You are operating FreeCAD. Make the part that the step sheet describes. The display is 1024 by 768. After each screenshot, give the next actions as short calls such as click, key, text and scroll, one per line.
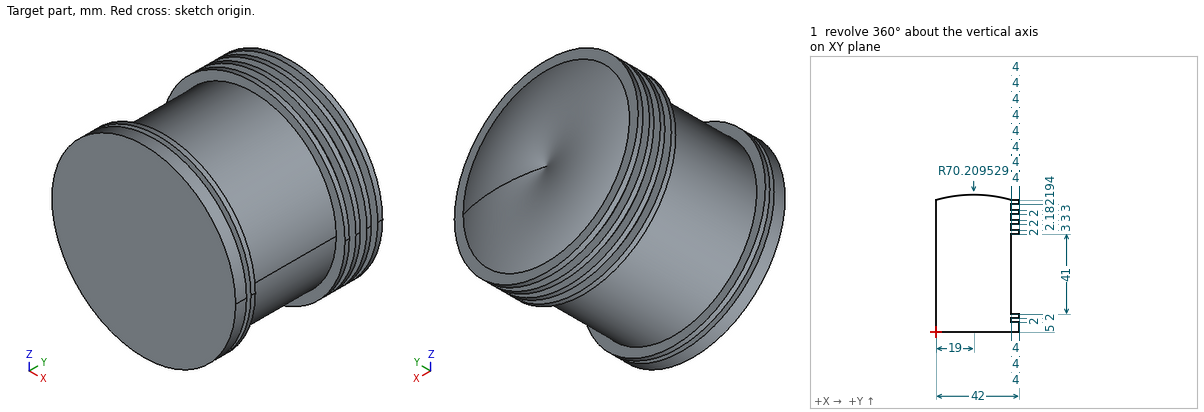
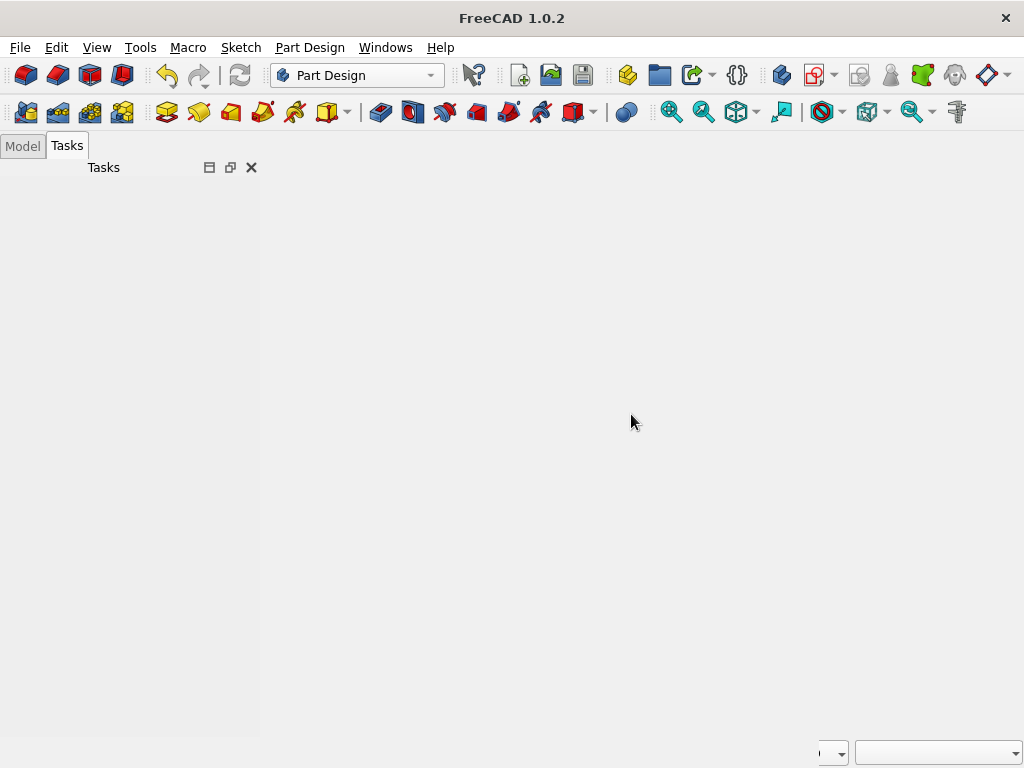
key(ctrl+n)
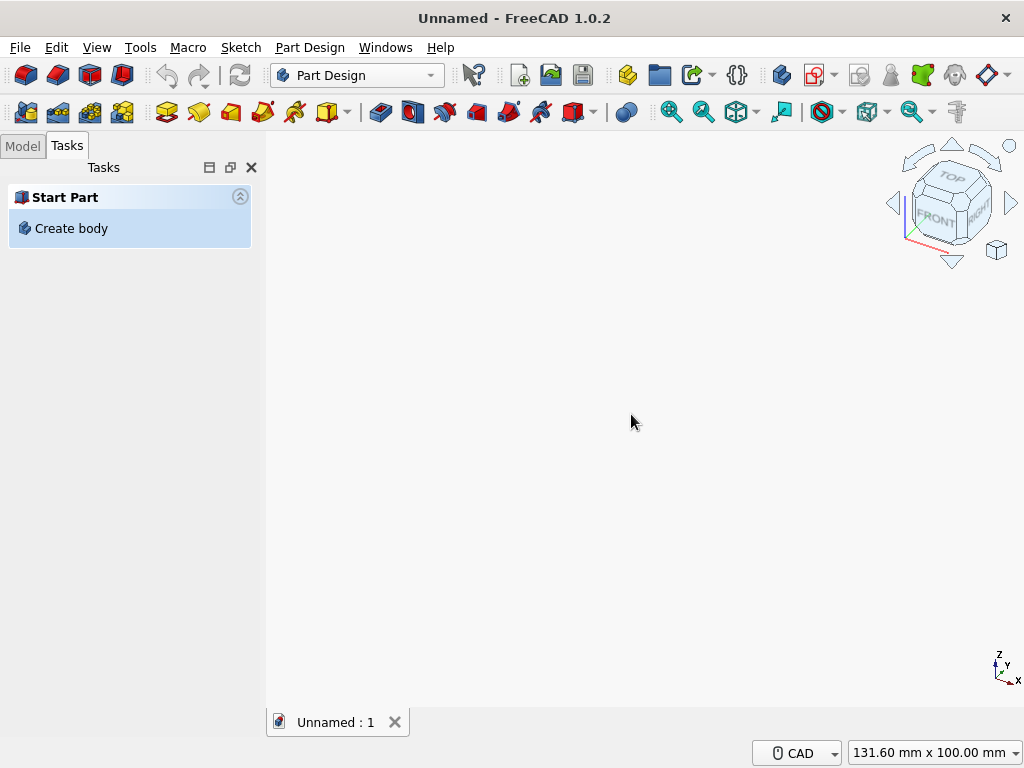
click(814, 76)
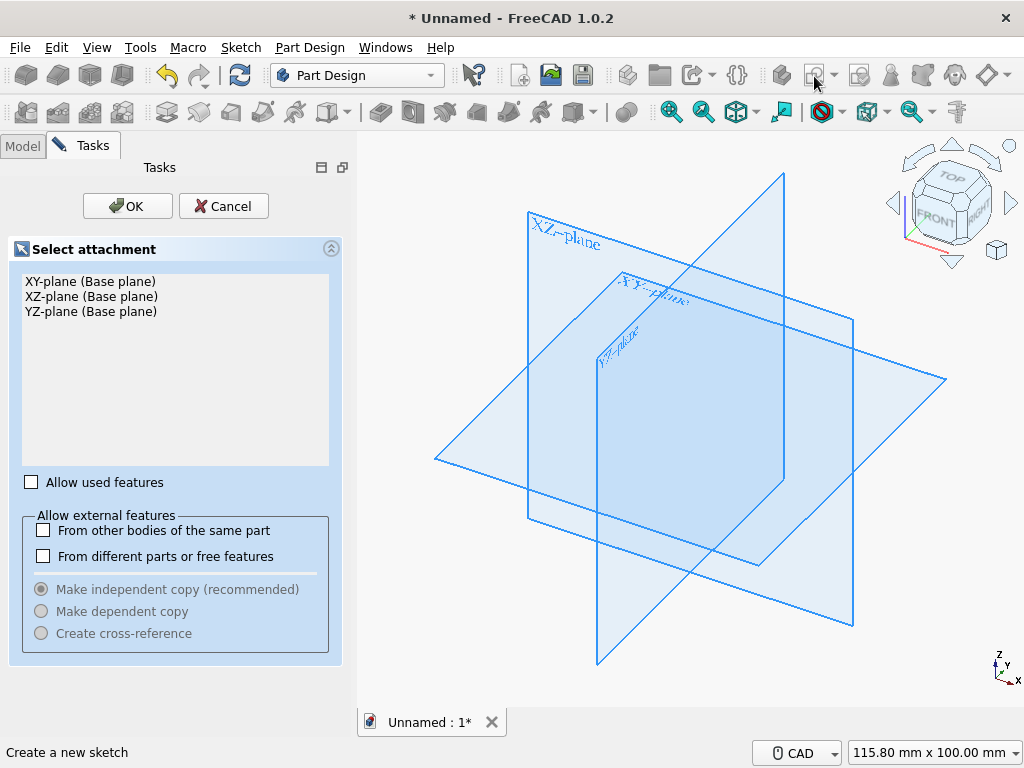
click(82, 282)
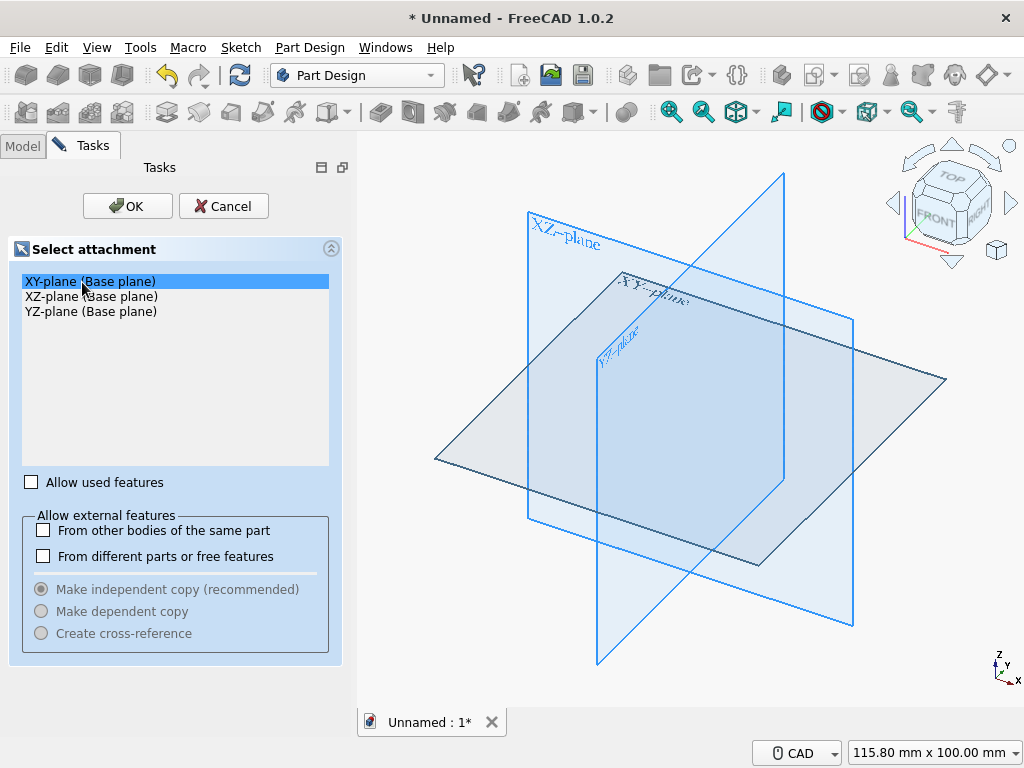
click(128, 206)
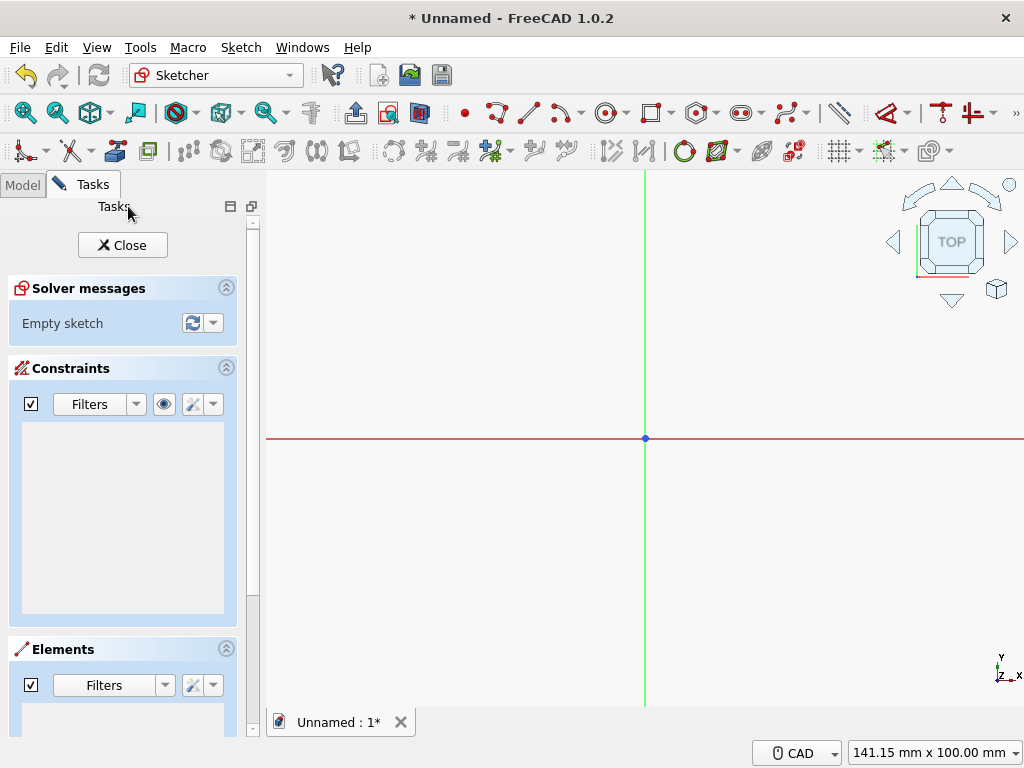
scroll(294, 679, down, 2)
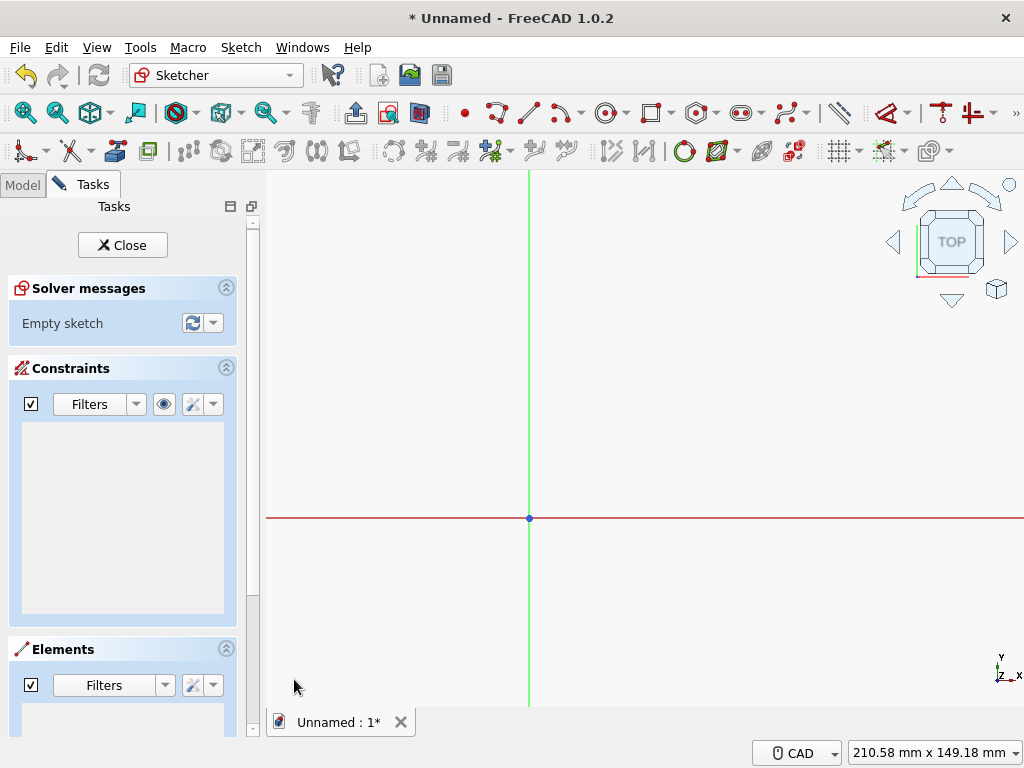
scroll(663, 299, up, 2)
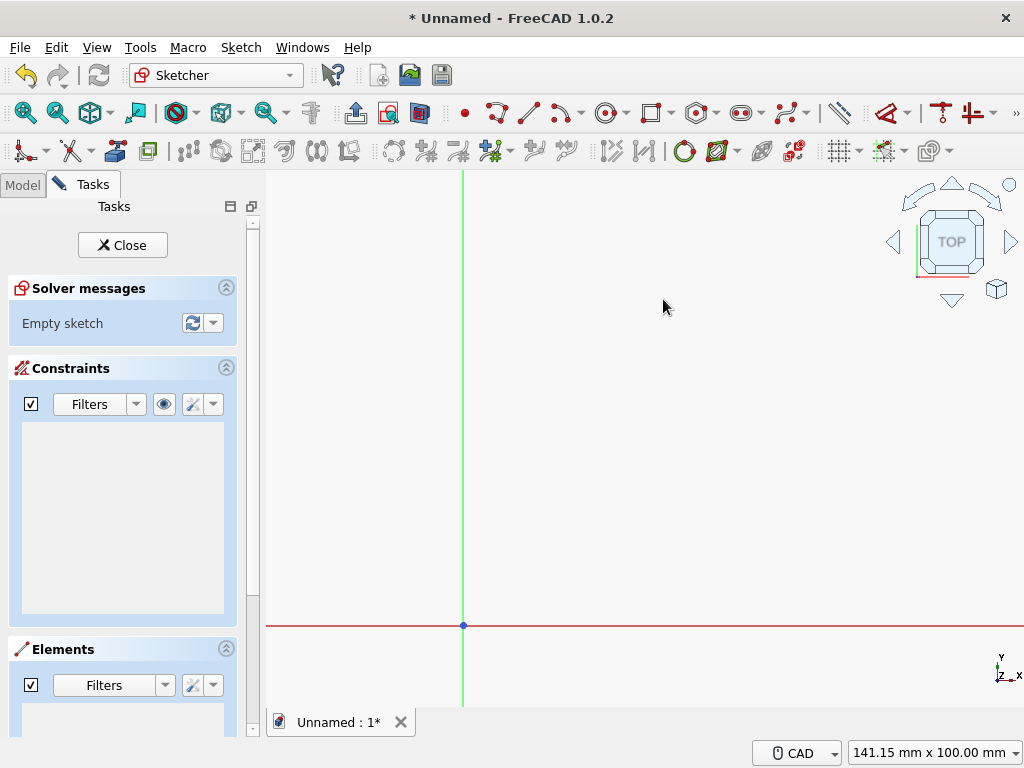
click(498, 114)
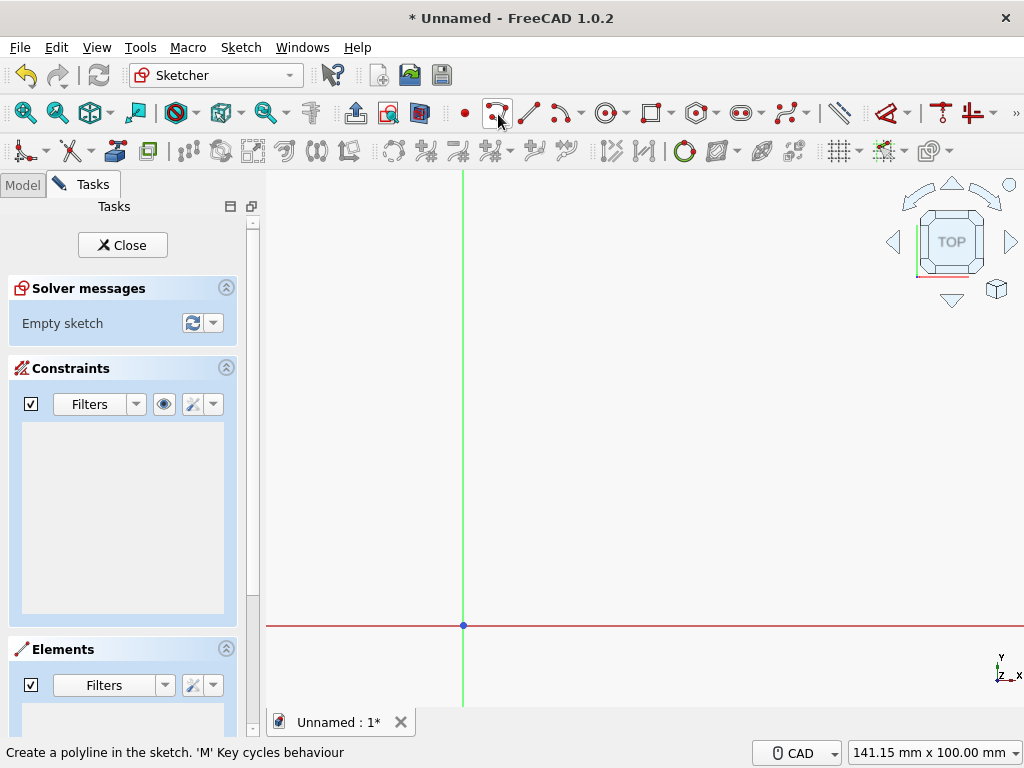
click(463, 265)
click(463, 626)
click(689, 617)
click(689, 599)
click(667, 599)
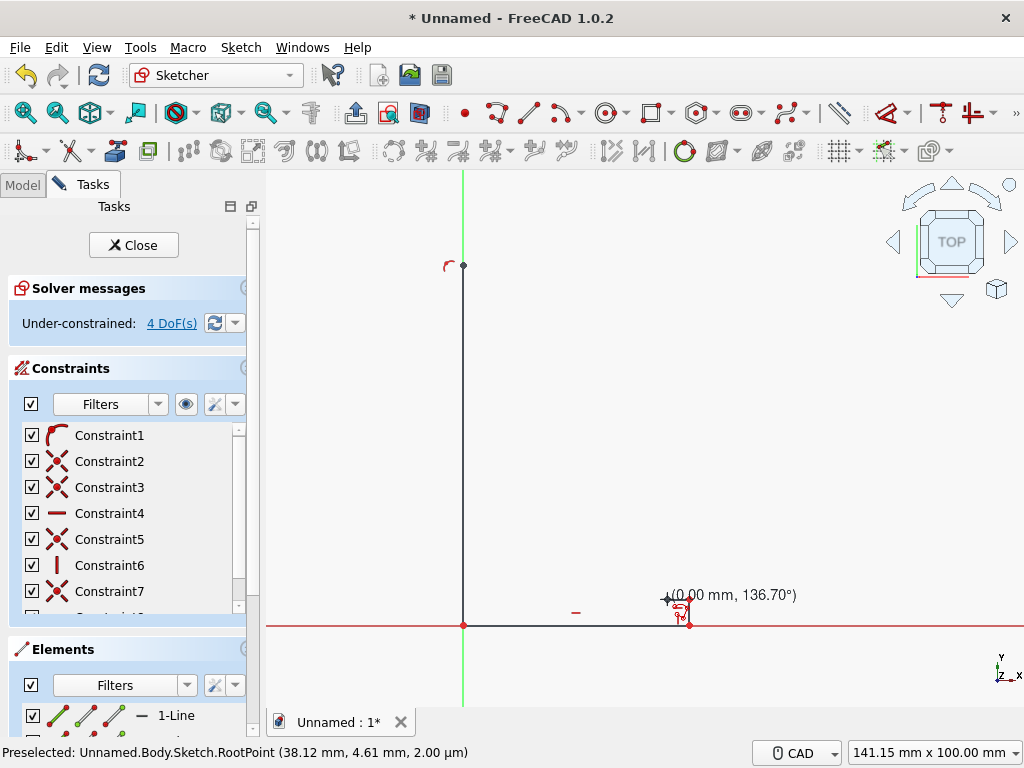
scroll(667, 588, up, 2)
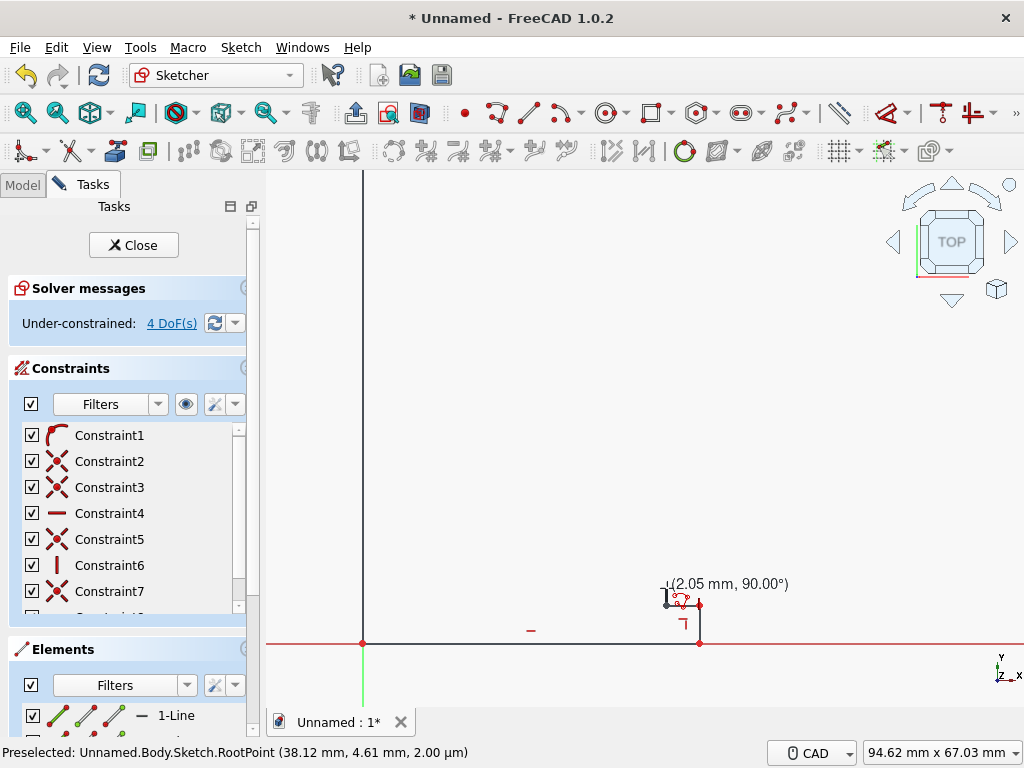
click(667, 588)
click(699, 588)
click(699, 572)
click(667, 572)
click(667, 243)
click(699, 243)
click(699, 227)
click(667, 227)
click(667, 203)
click(699, 203)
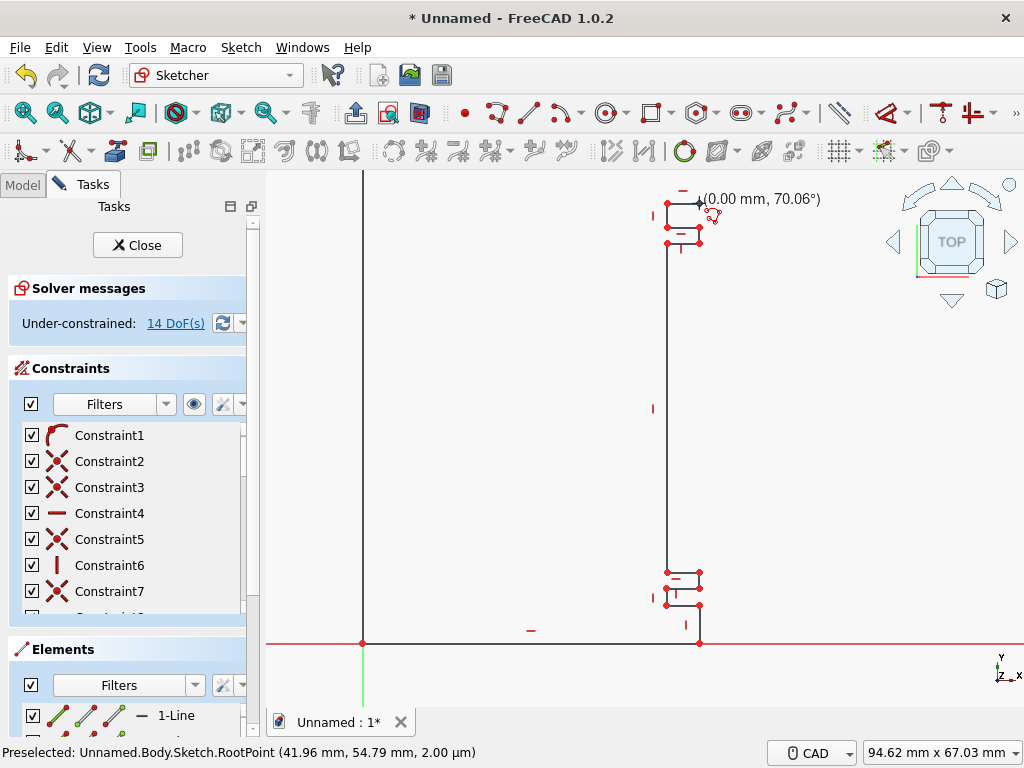
scroll(669, 589, down, 2)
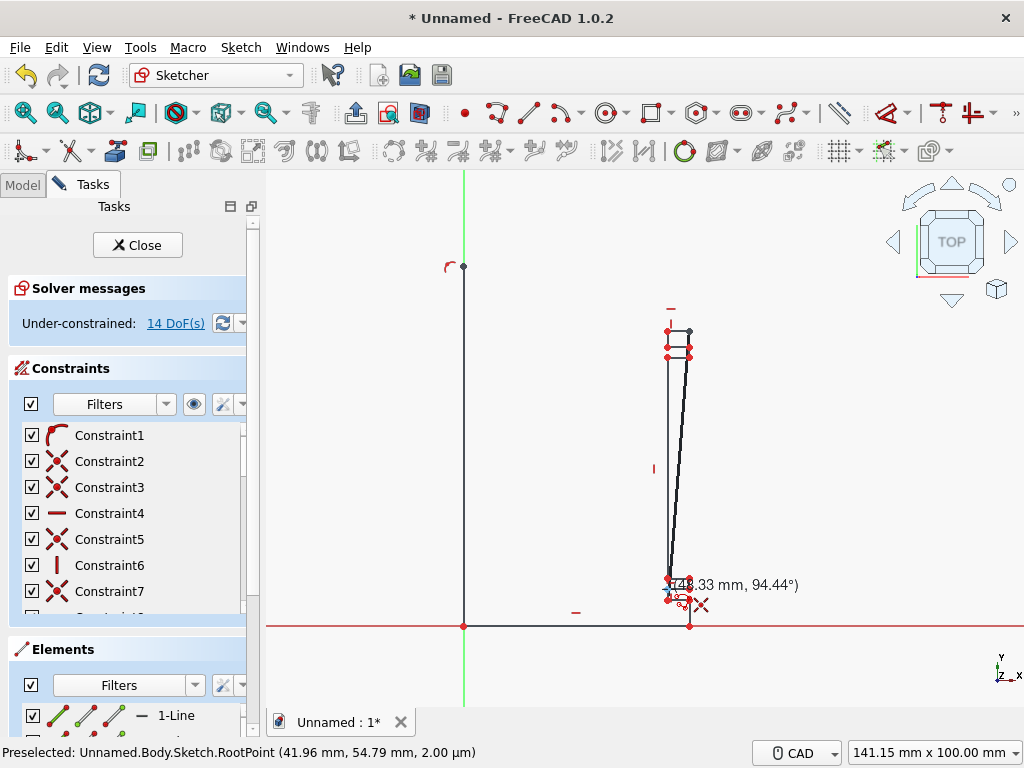
scroll(689, 320, up, 2)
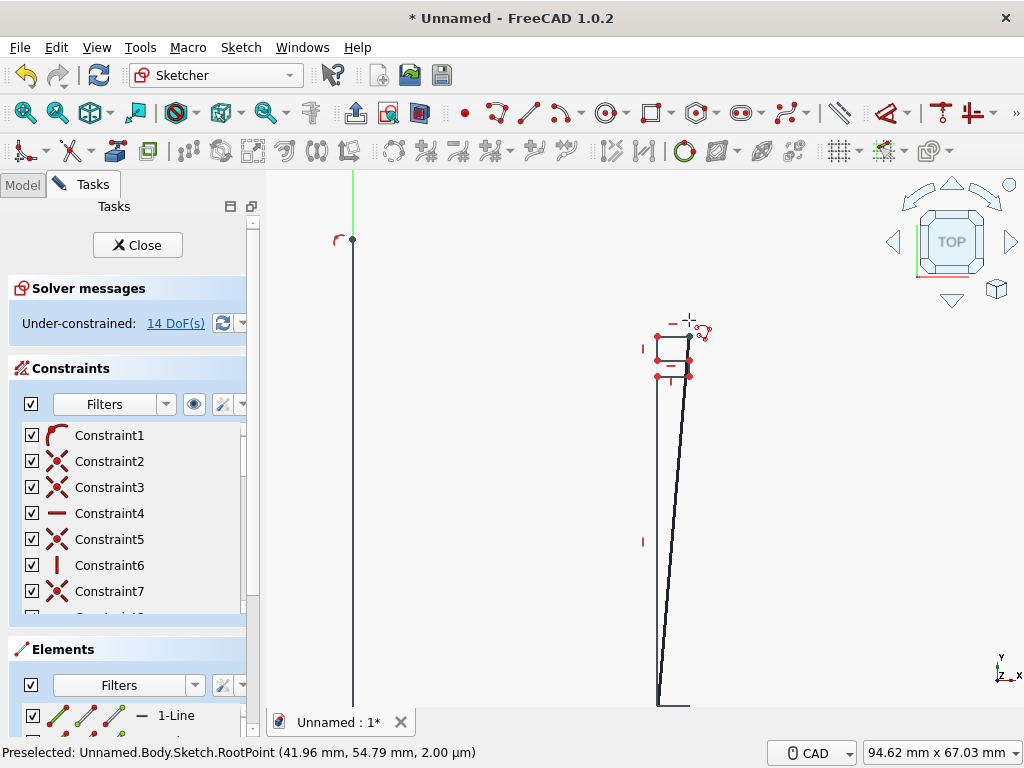
click(689, 320)
click(657, 320)
click(657, 296)
click(689, 296)
click(689, 280)
click(657, 280)
click(657, 256)
click(689, 256)
click(689, 238)
click(657, 238)
right_click(657, 238)